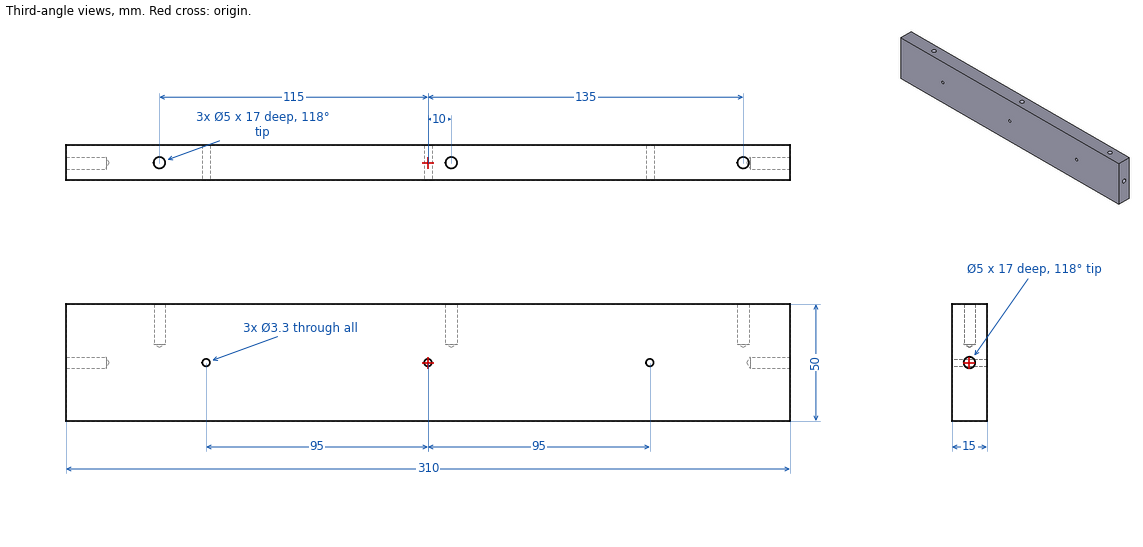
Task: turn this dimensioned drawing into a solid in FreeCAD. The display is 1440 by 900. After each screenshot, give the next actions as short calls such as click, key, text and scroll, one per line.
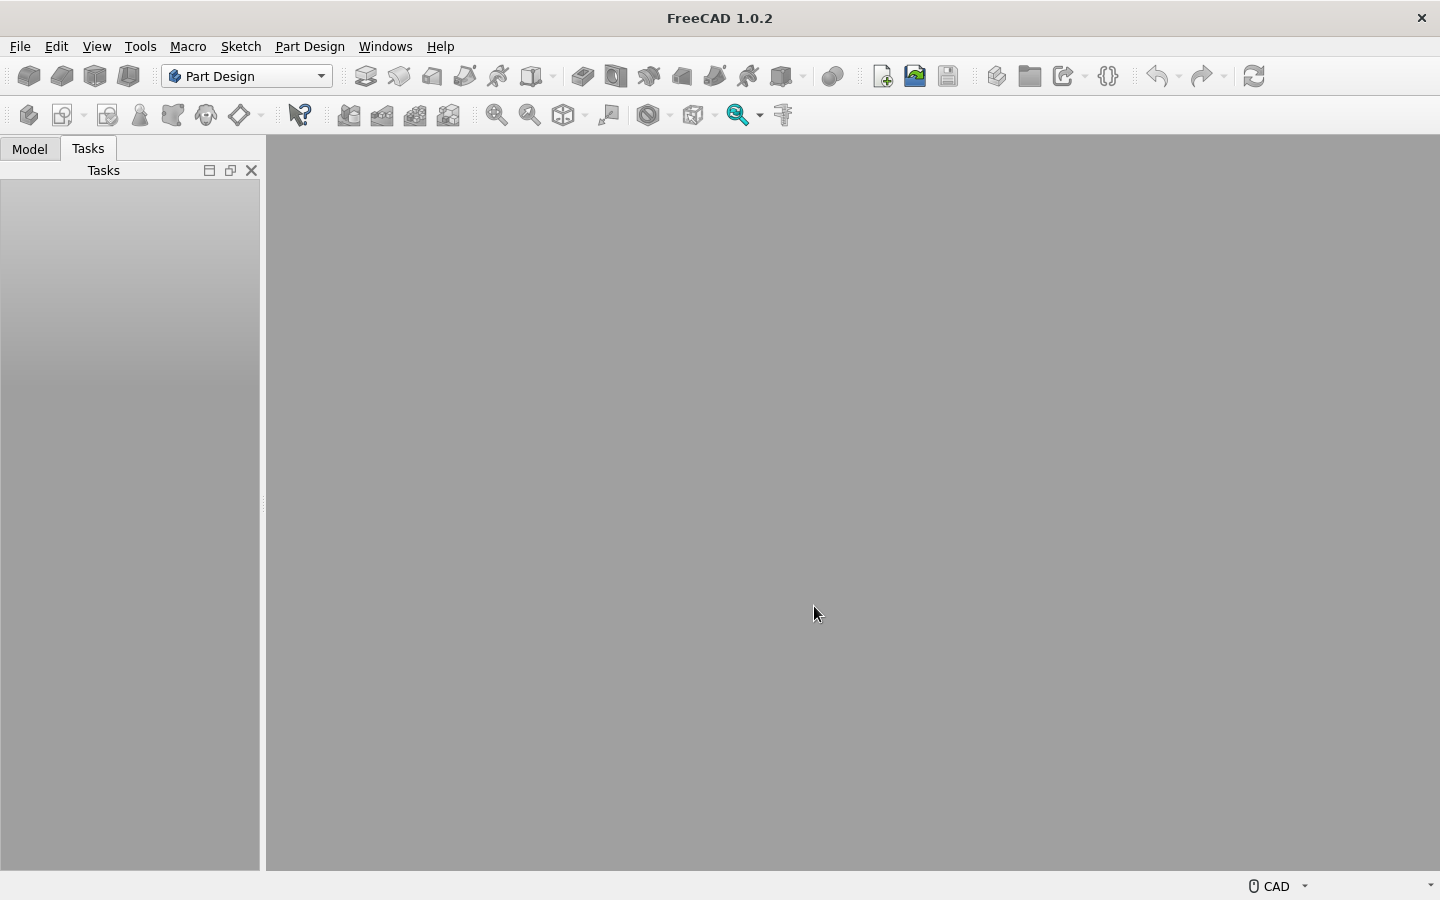
click(882, 76)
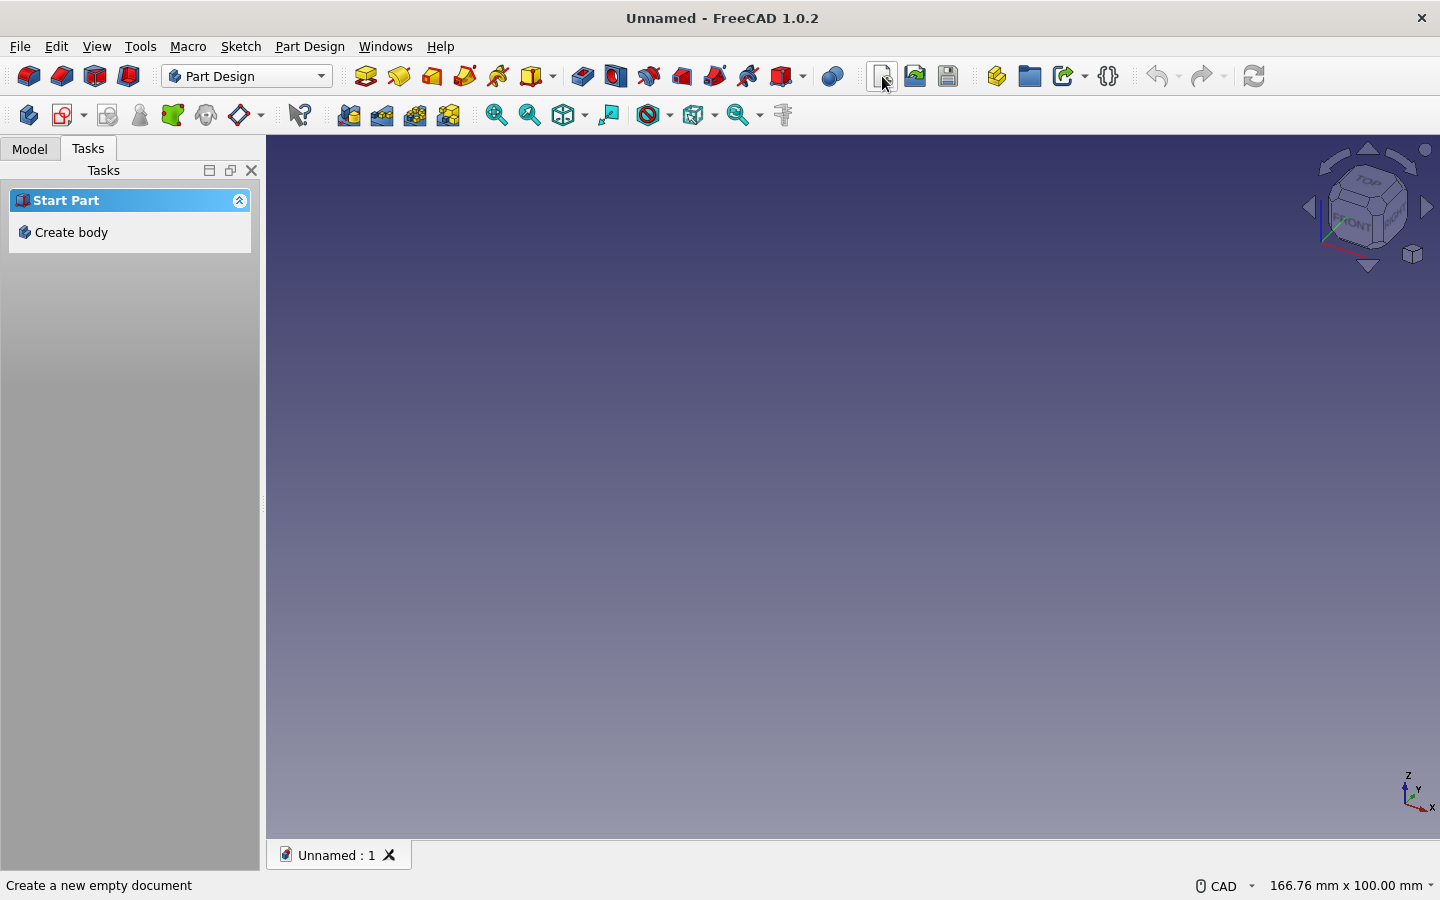
click(62, 116)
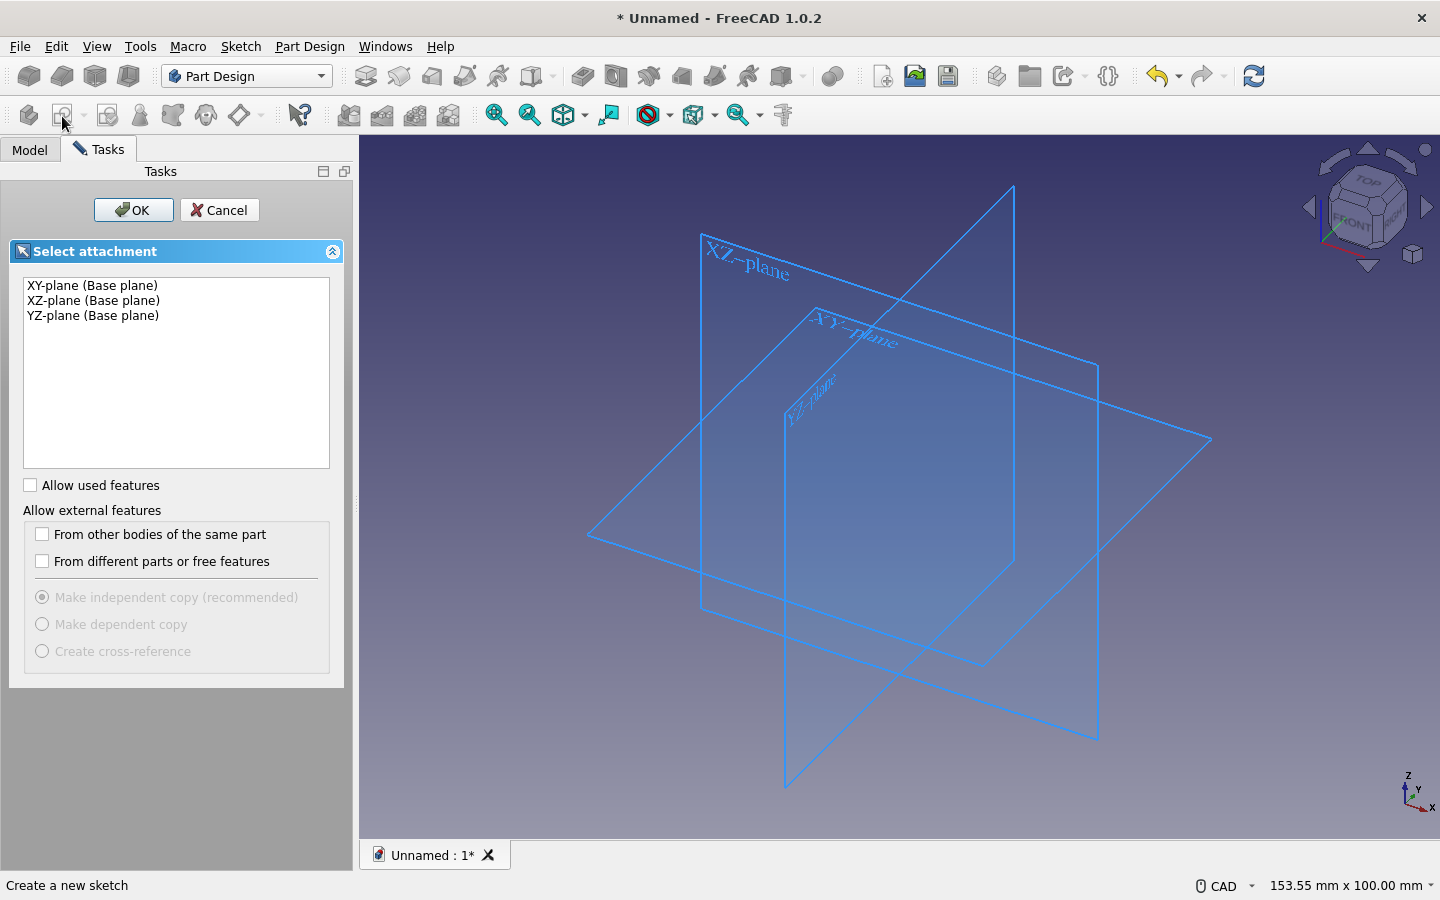
click(84, 300)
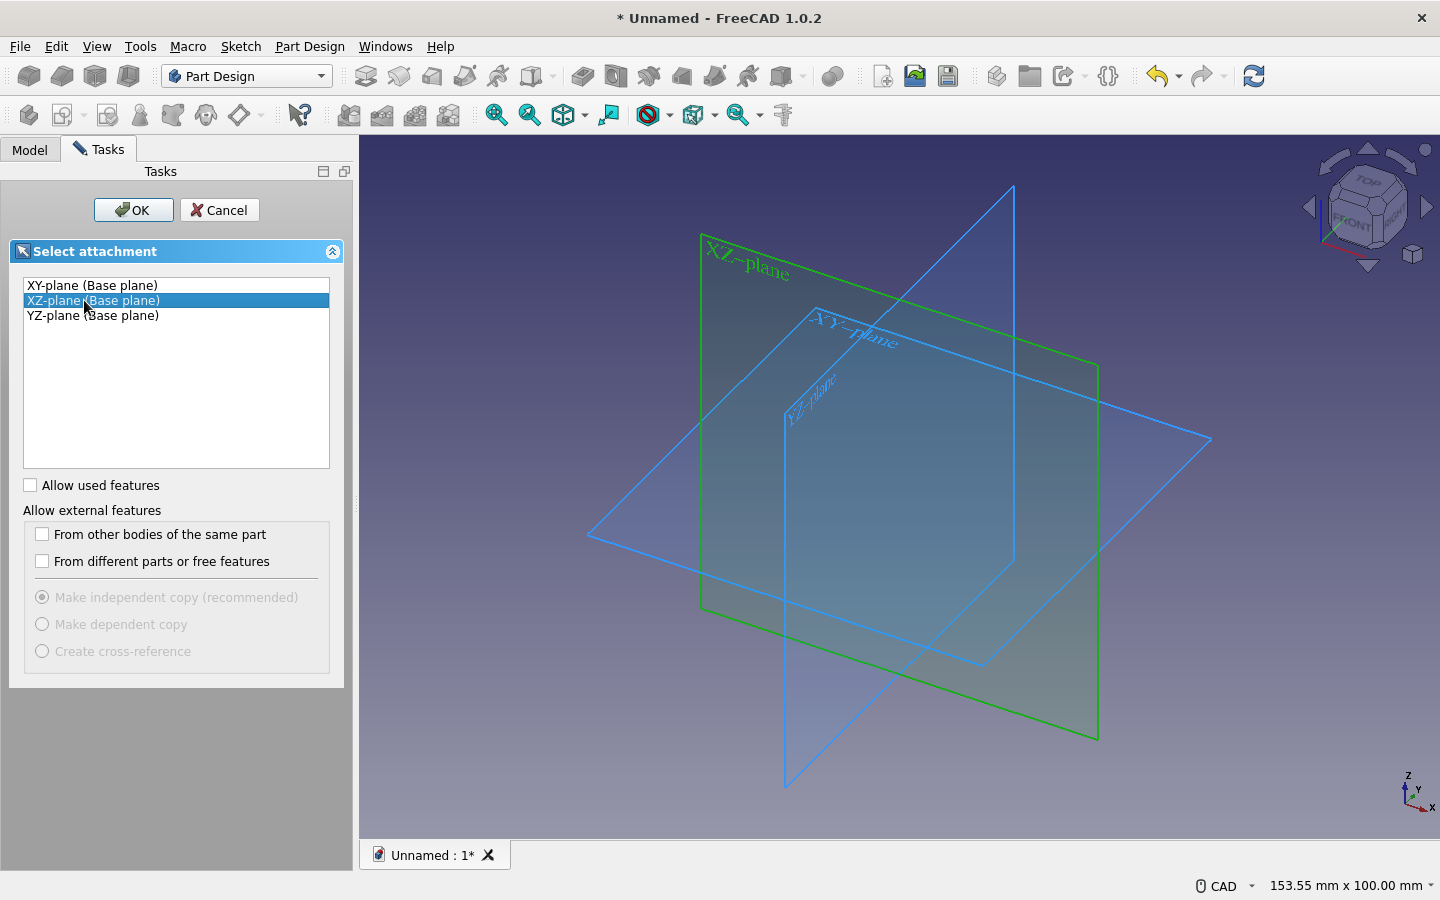
click(134, 210)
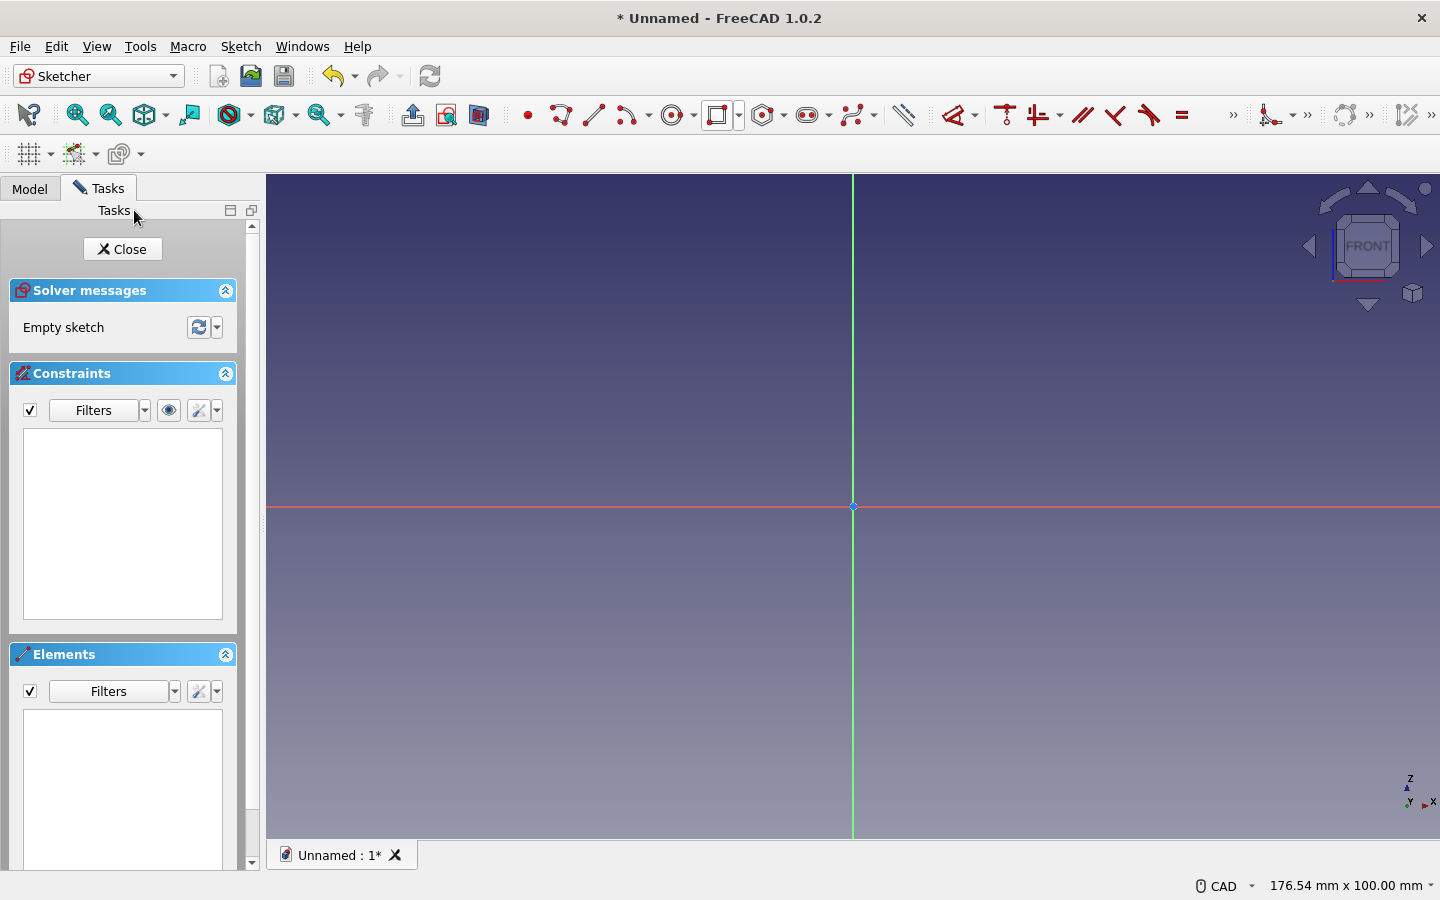
scroll(745, 506, down, 5)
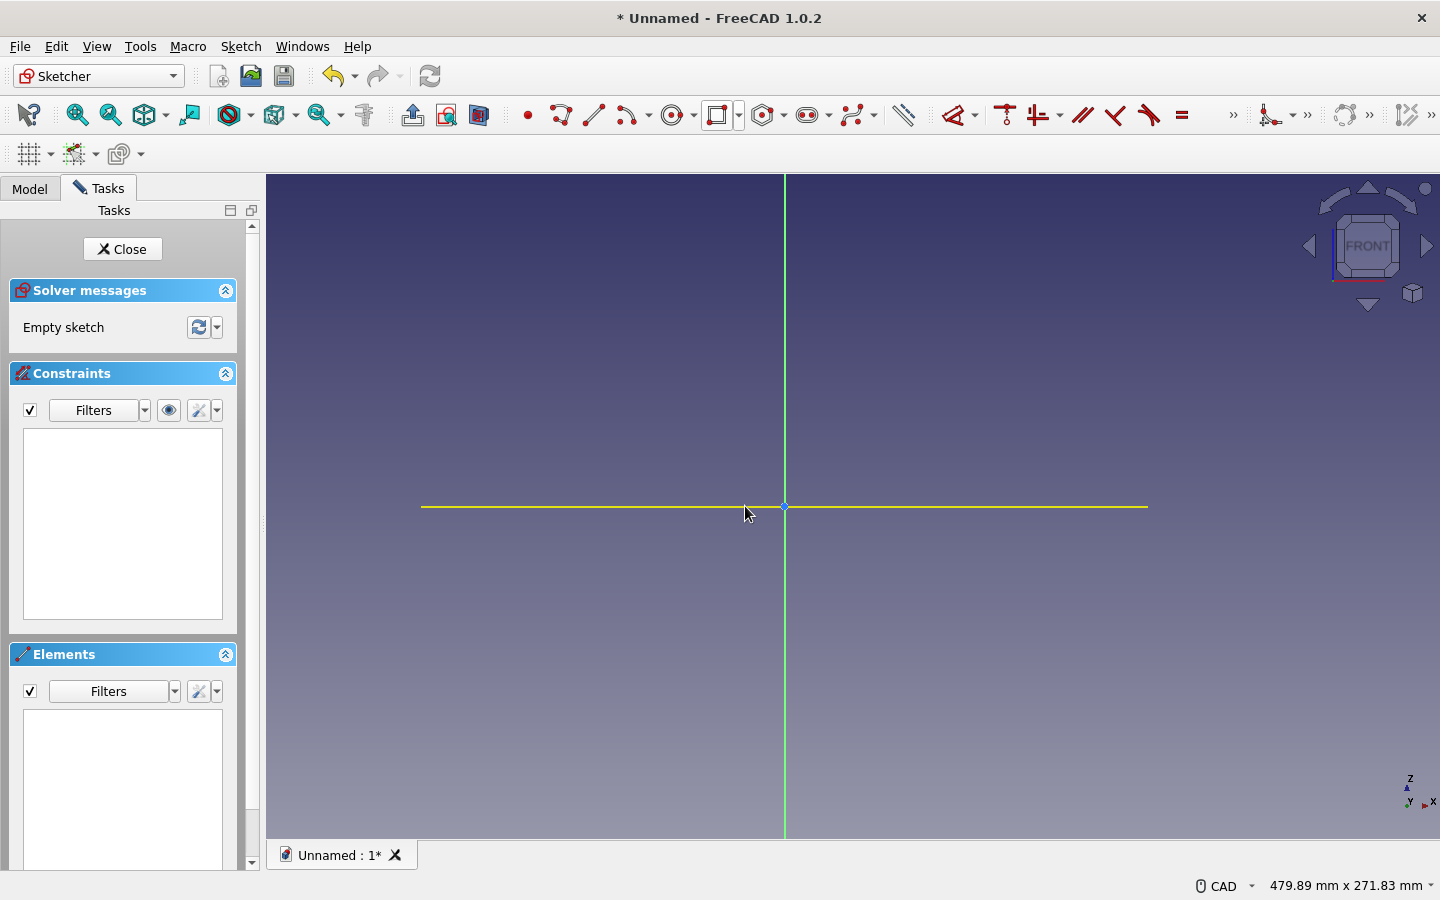
key(g)
key(v)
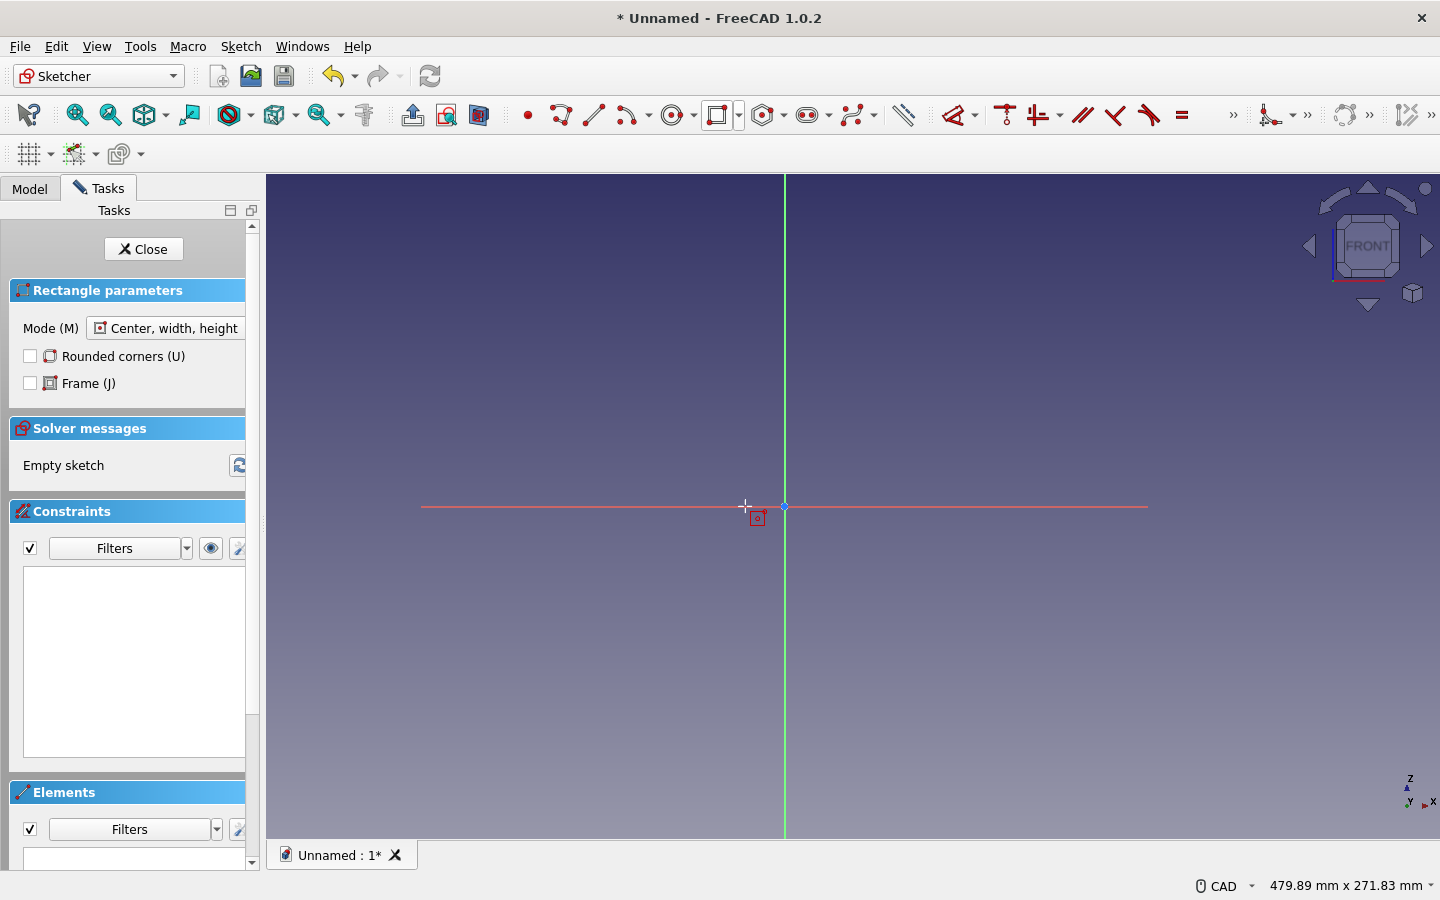
click(785, 506)
click(1164, 445)
key(Escape)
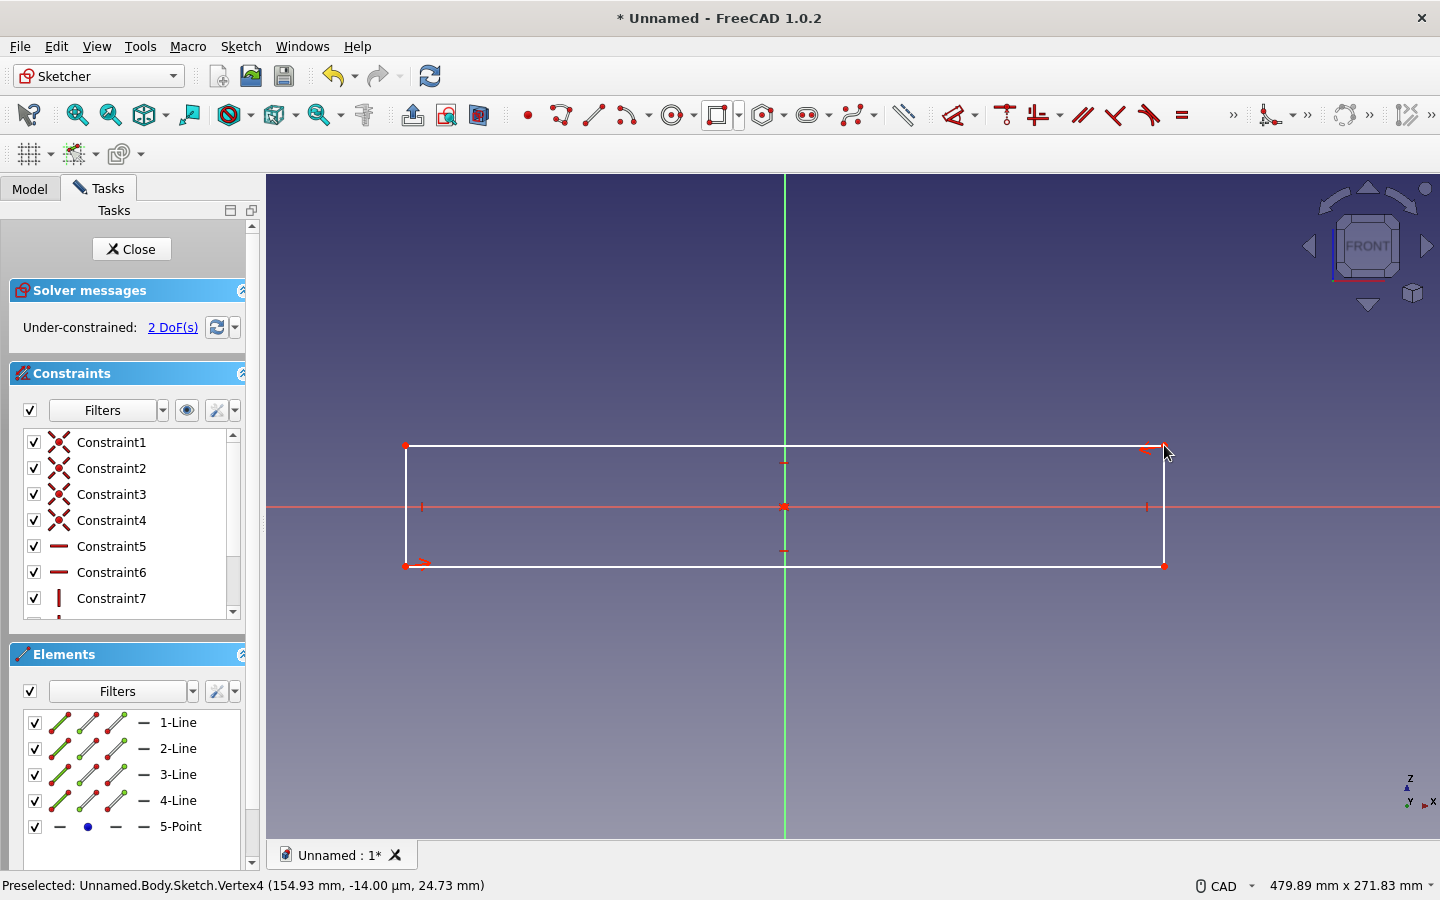
click(952, 116)